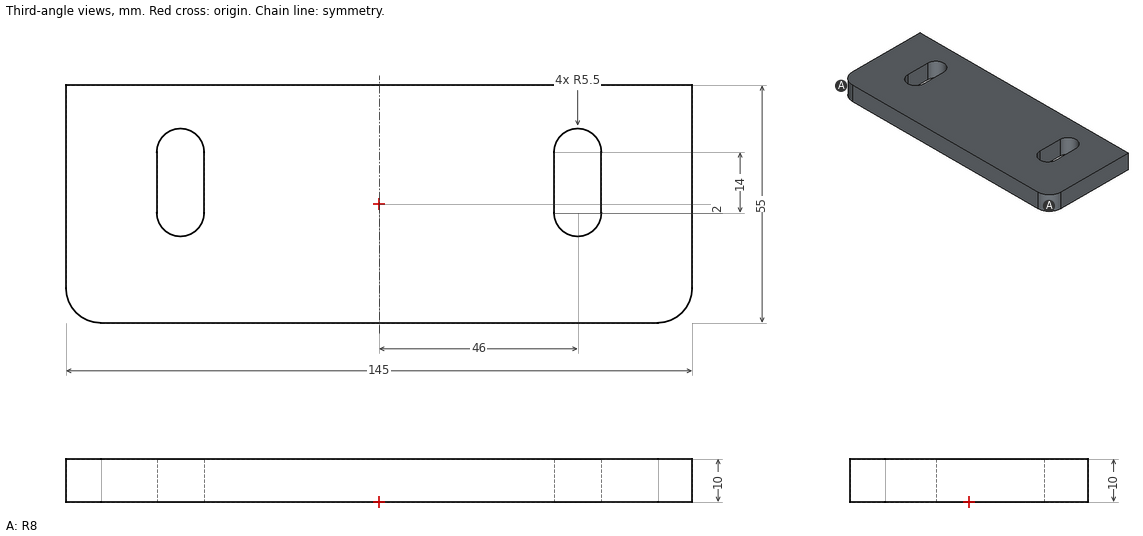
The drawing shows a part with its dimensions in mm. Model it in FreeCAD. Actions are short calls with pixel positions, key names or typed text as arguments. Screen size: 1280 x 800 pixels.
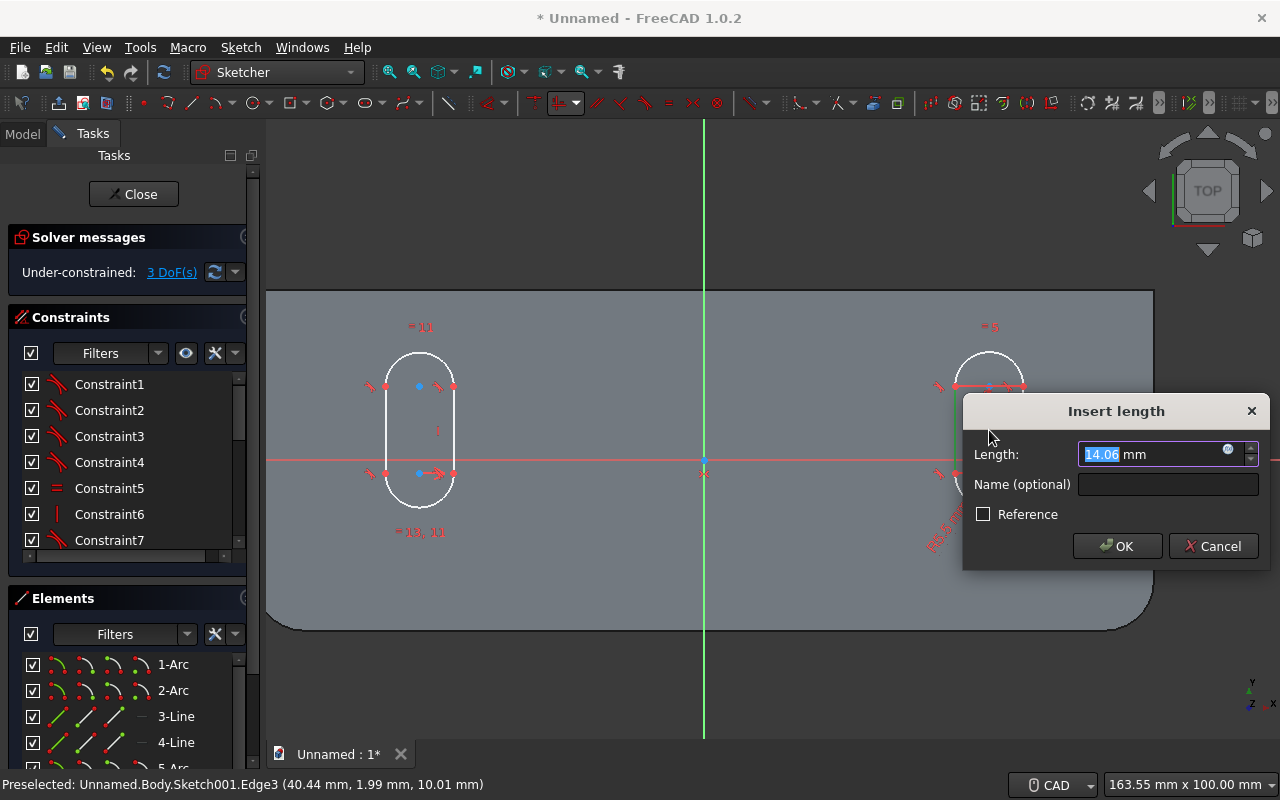
text(14)
key(Return)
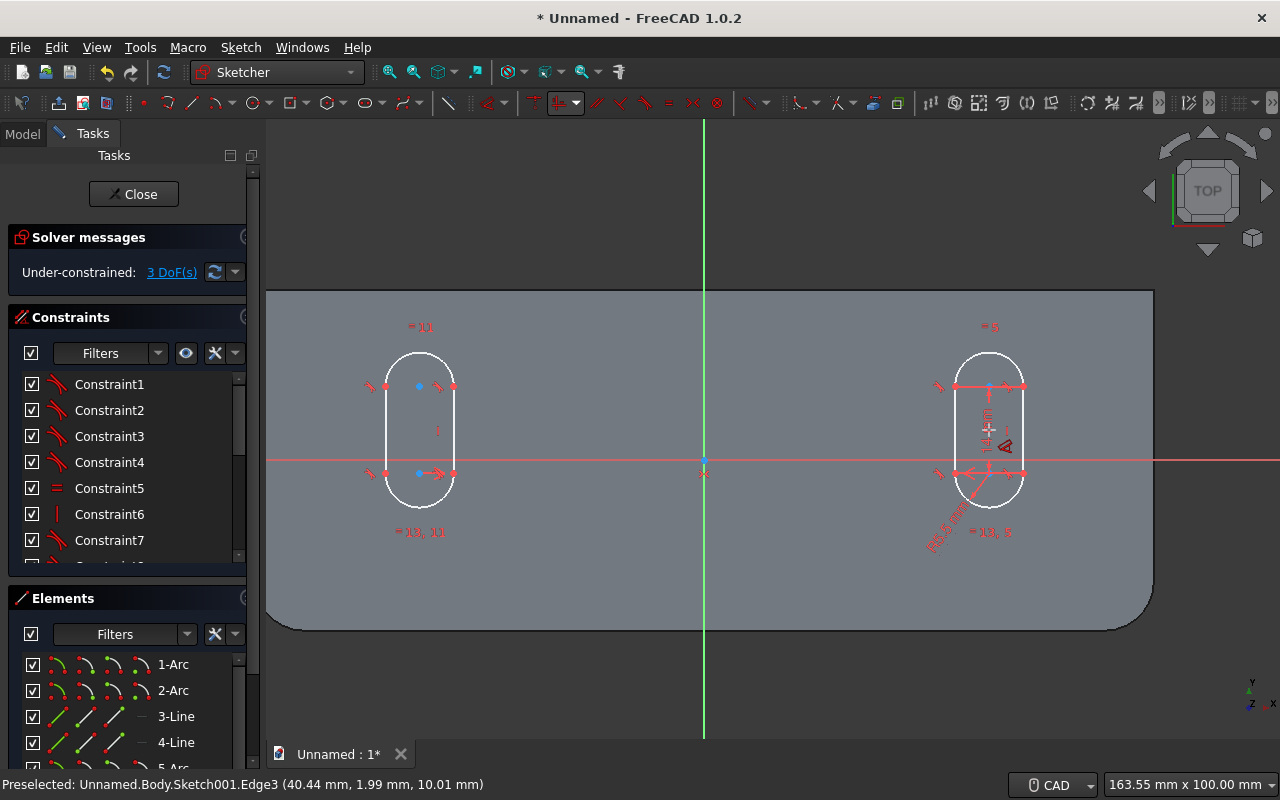
click(386, 447)
click(352, 430)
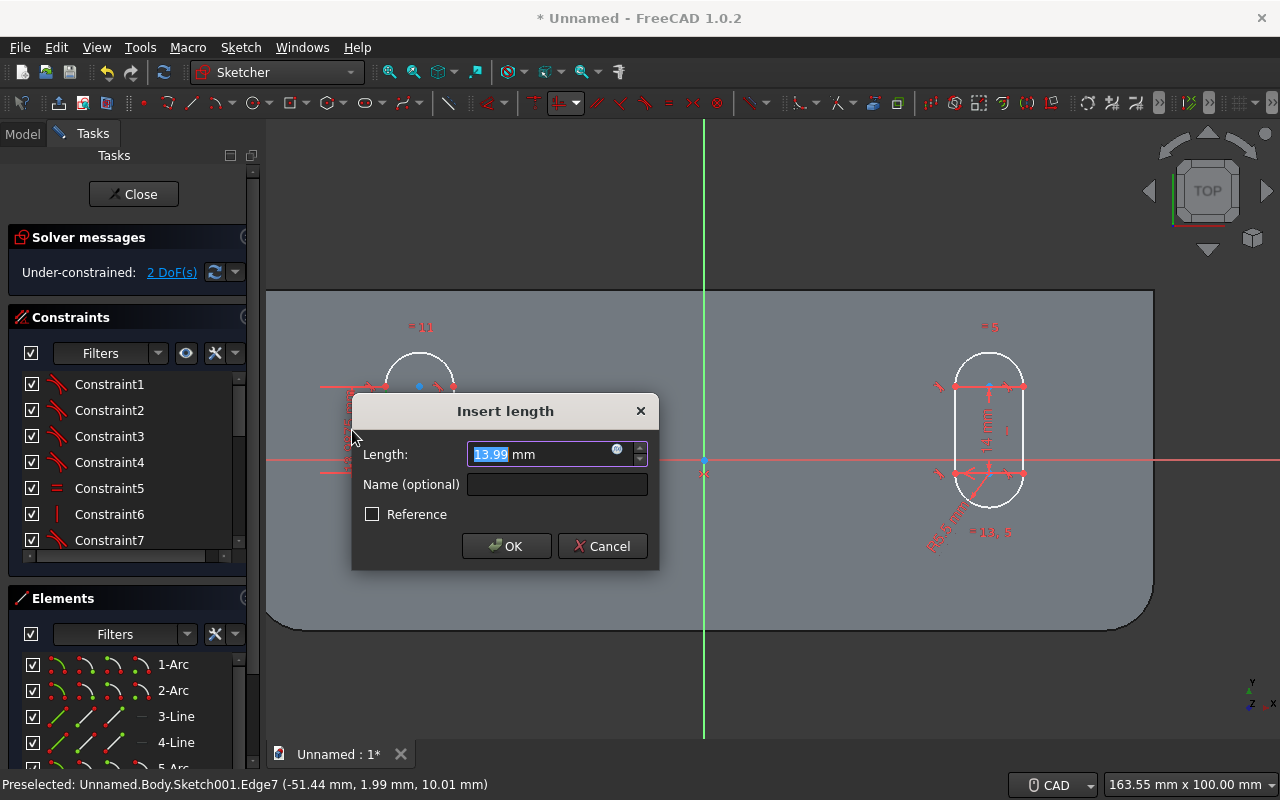
text(14)
key(Return)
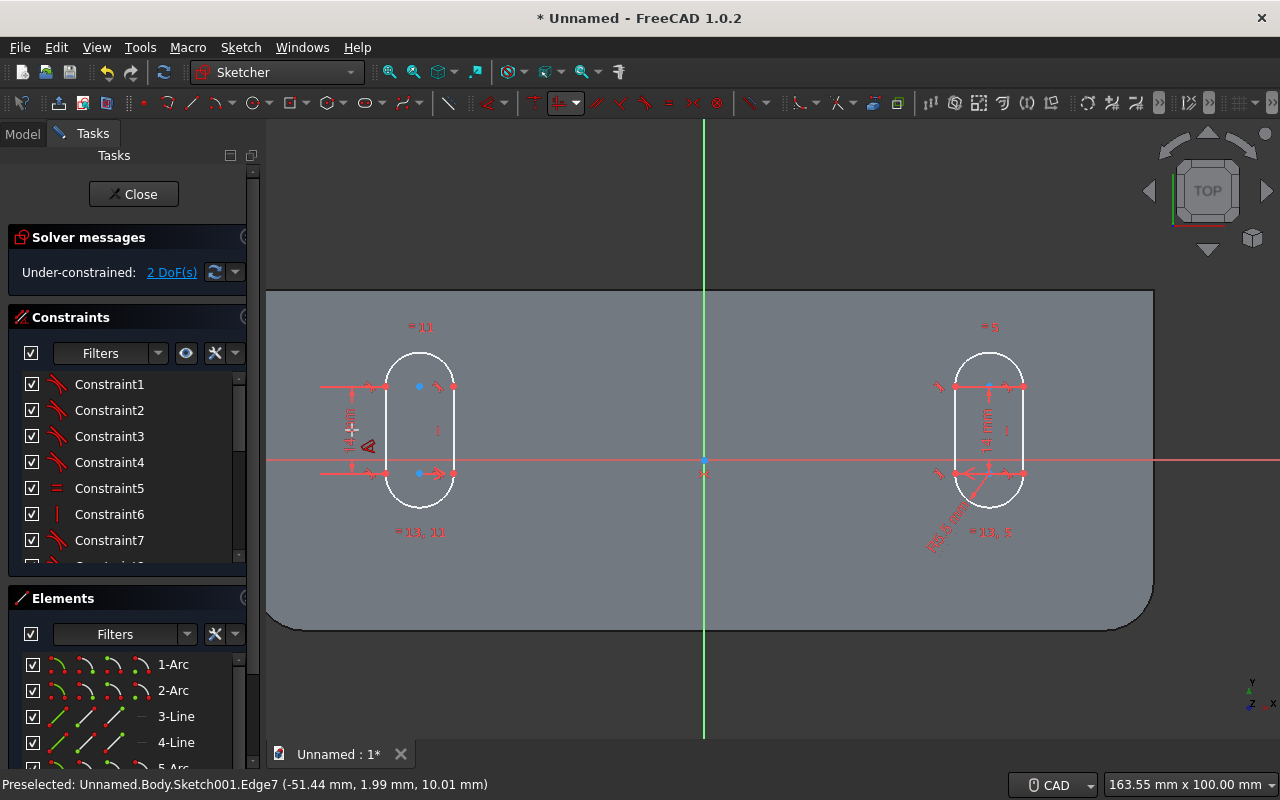
scroll(955, 474, up, 6)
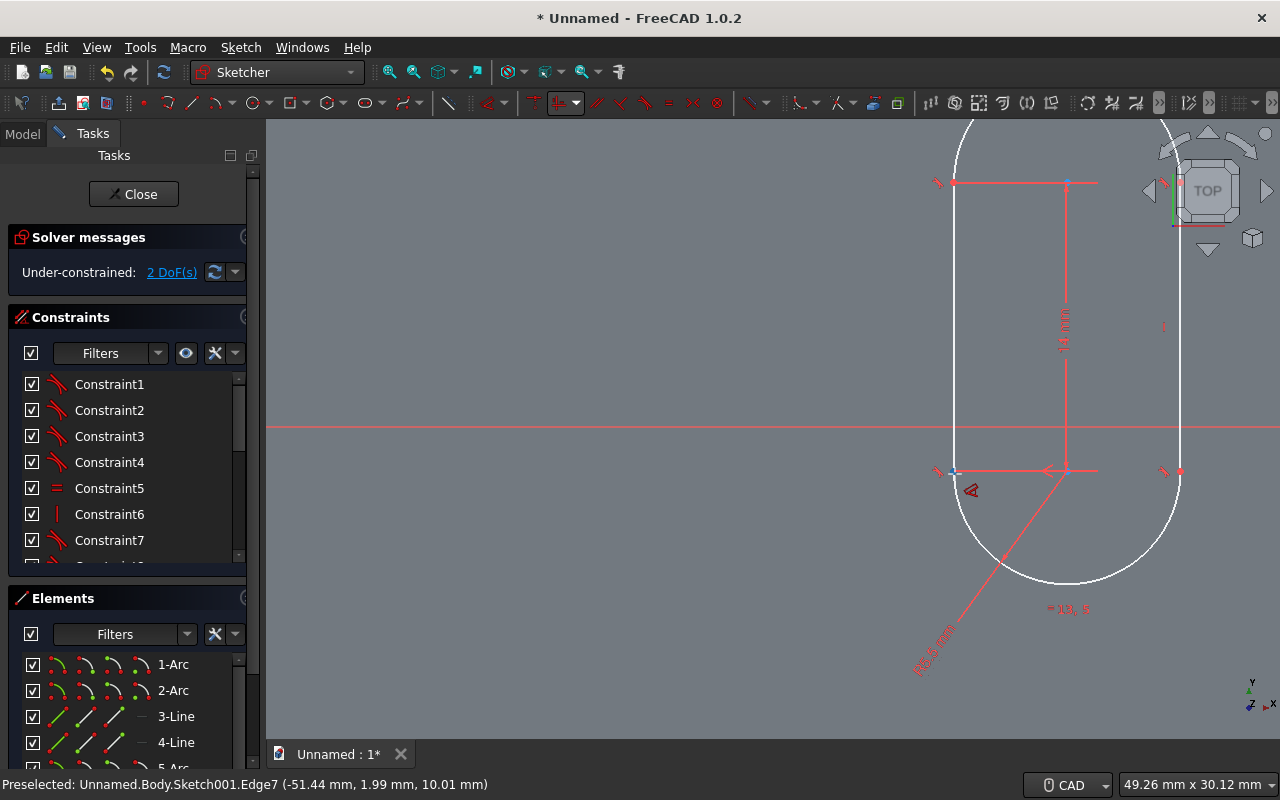
click(954, 471)
click(988, 449)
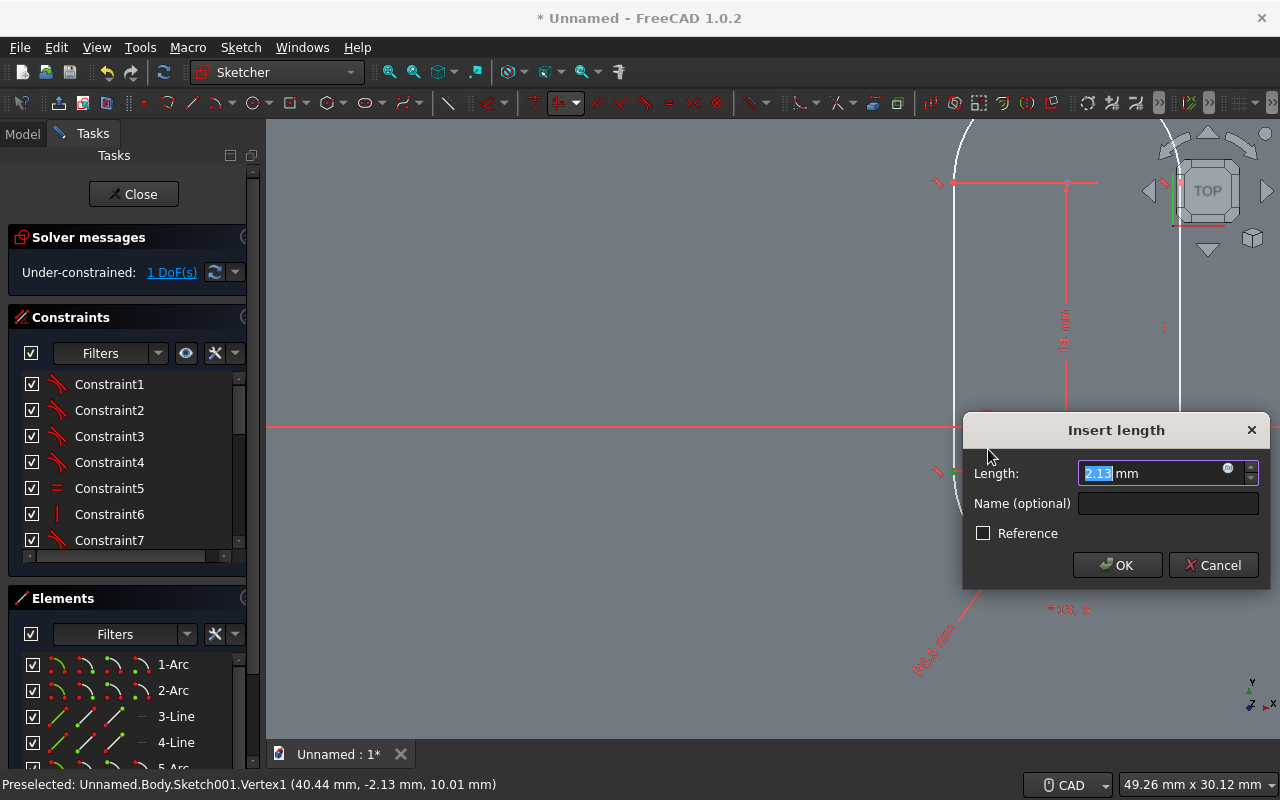
text(2)
key(Return)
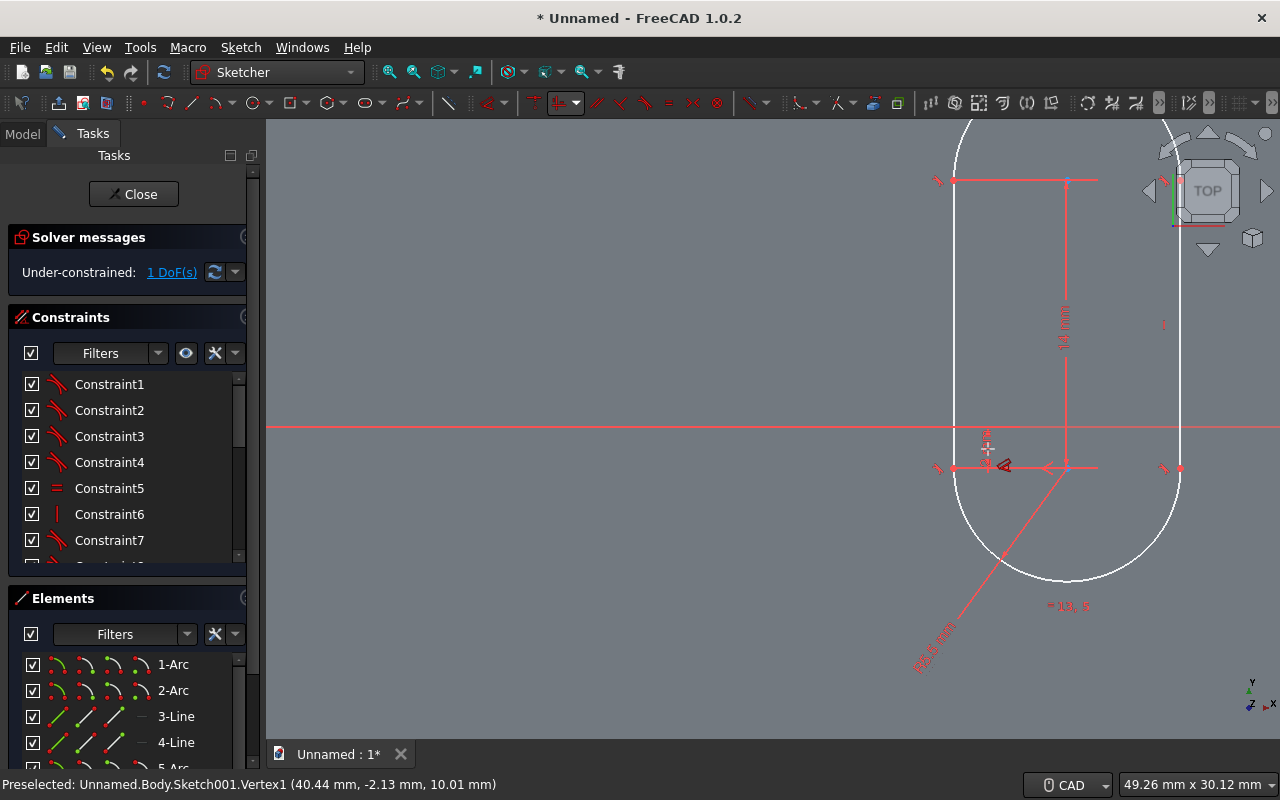
scroll(956, 474, down, 6)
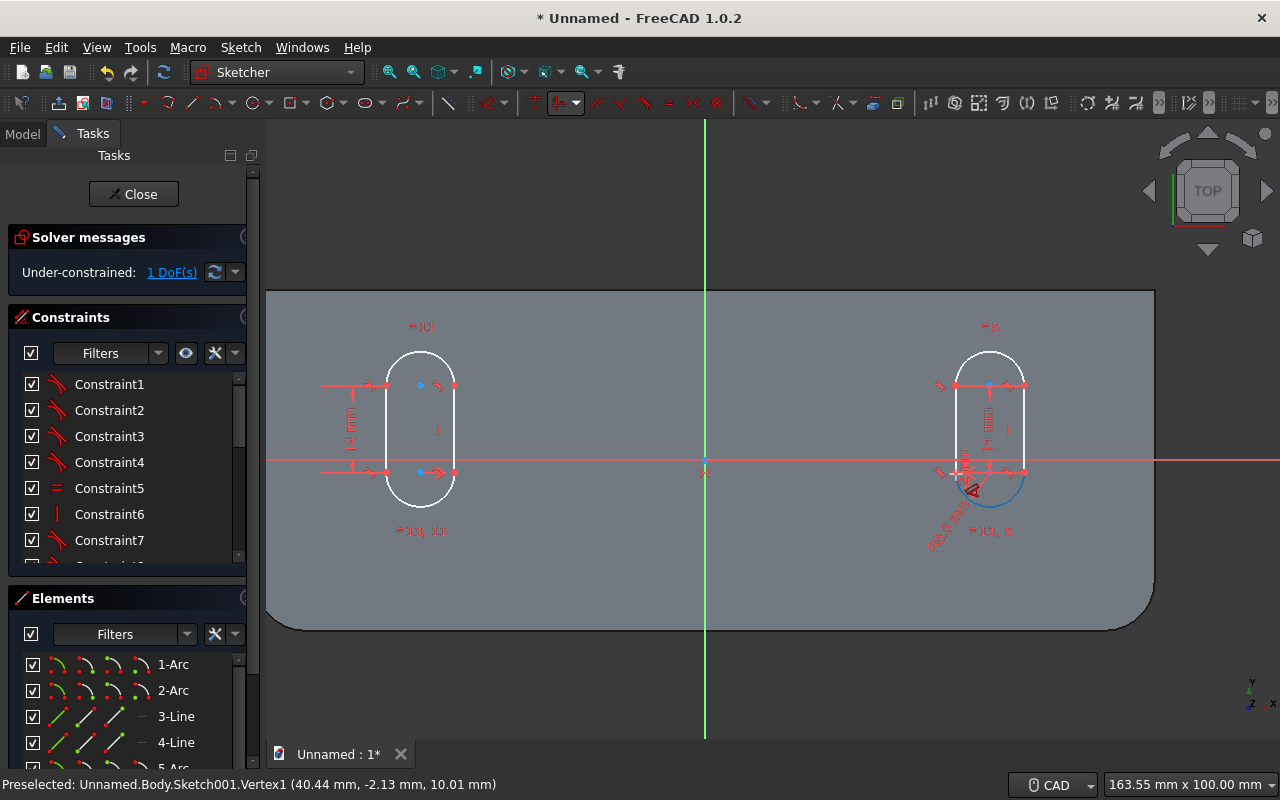
click(990, 473)
click(848, 507)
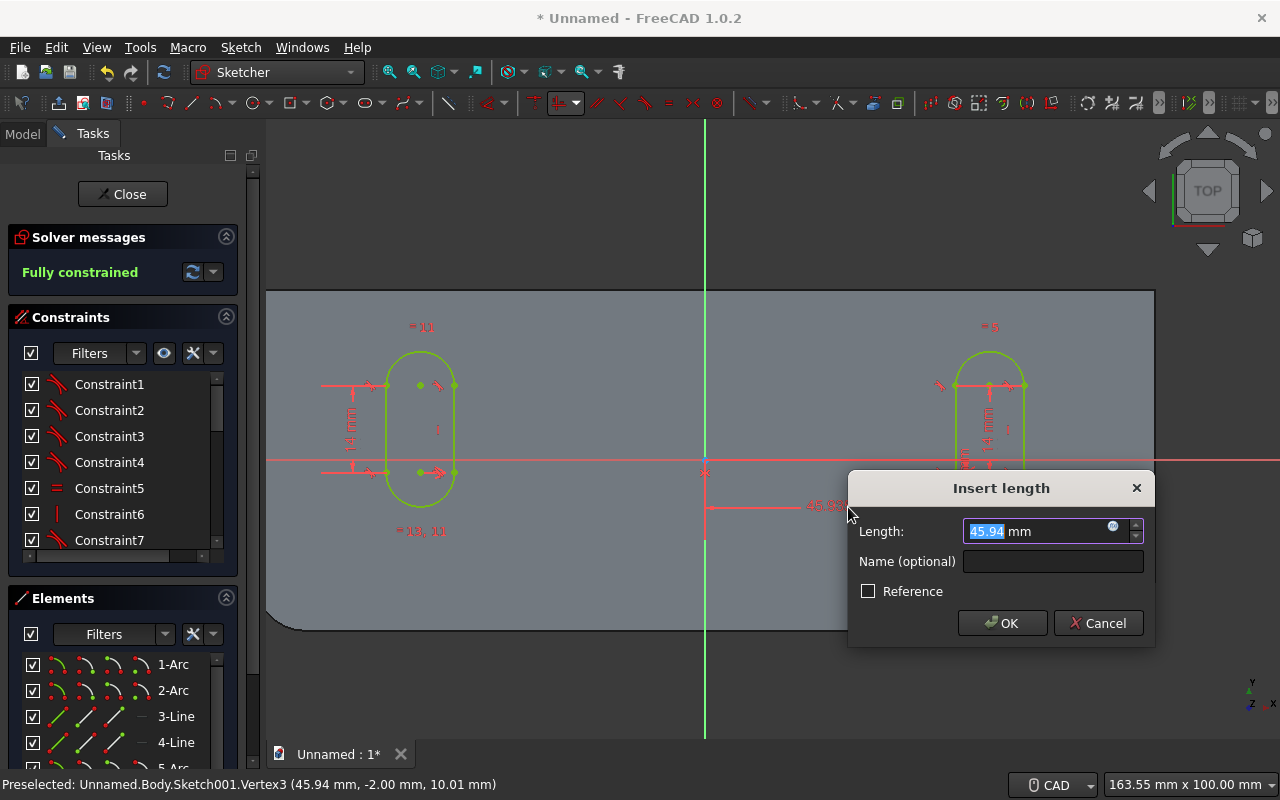
text(46)
key(Return)
key(Escape)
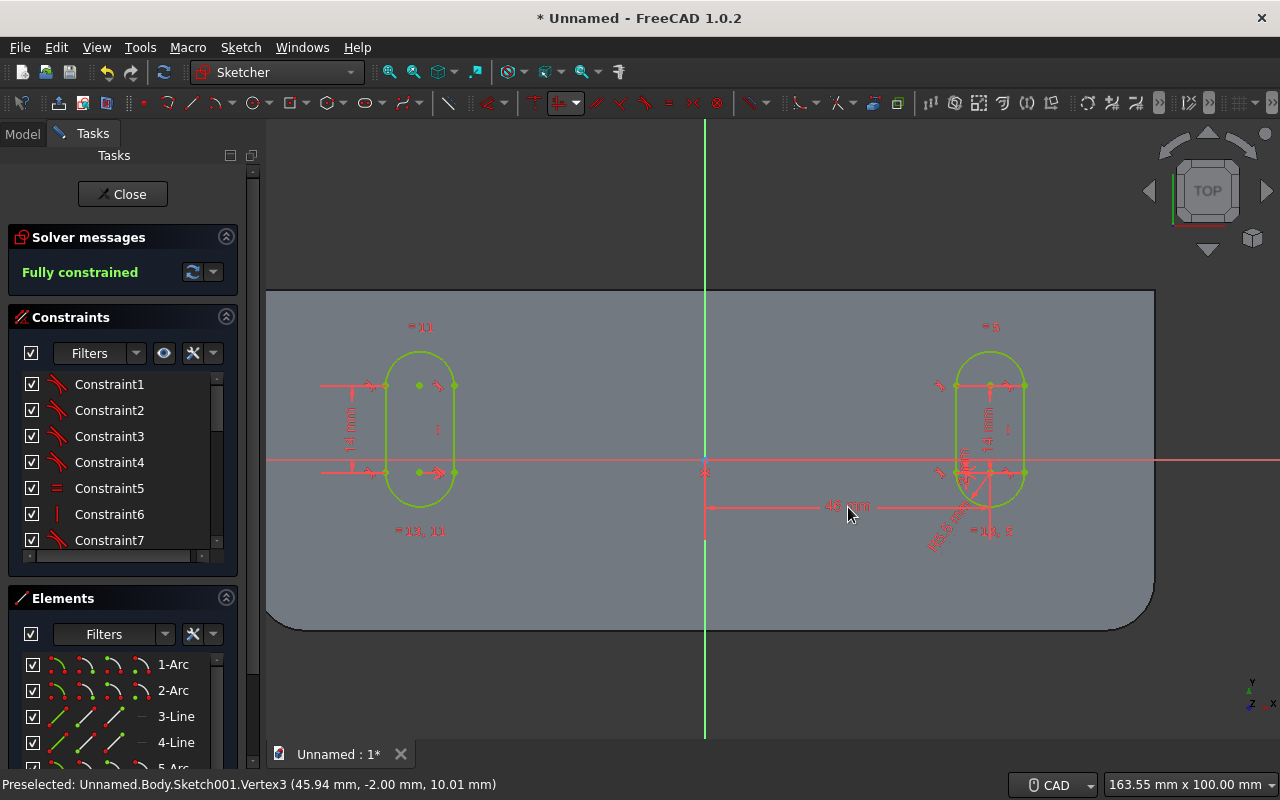
click(123, 194)